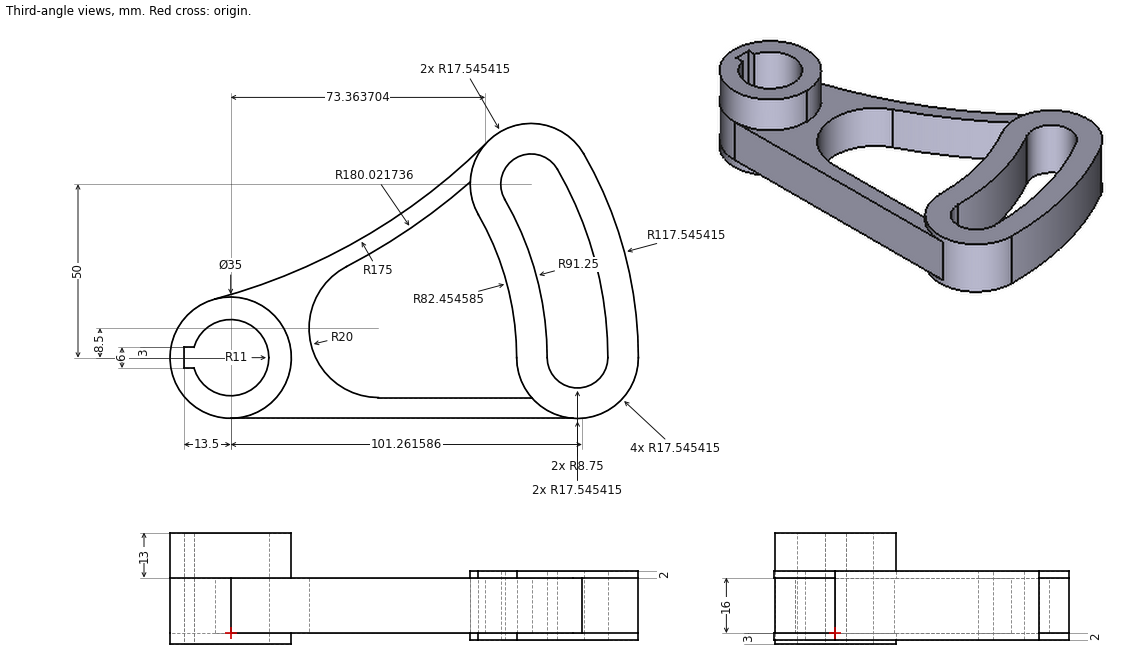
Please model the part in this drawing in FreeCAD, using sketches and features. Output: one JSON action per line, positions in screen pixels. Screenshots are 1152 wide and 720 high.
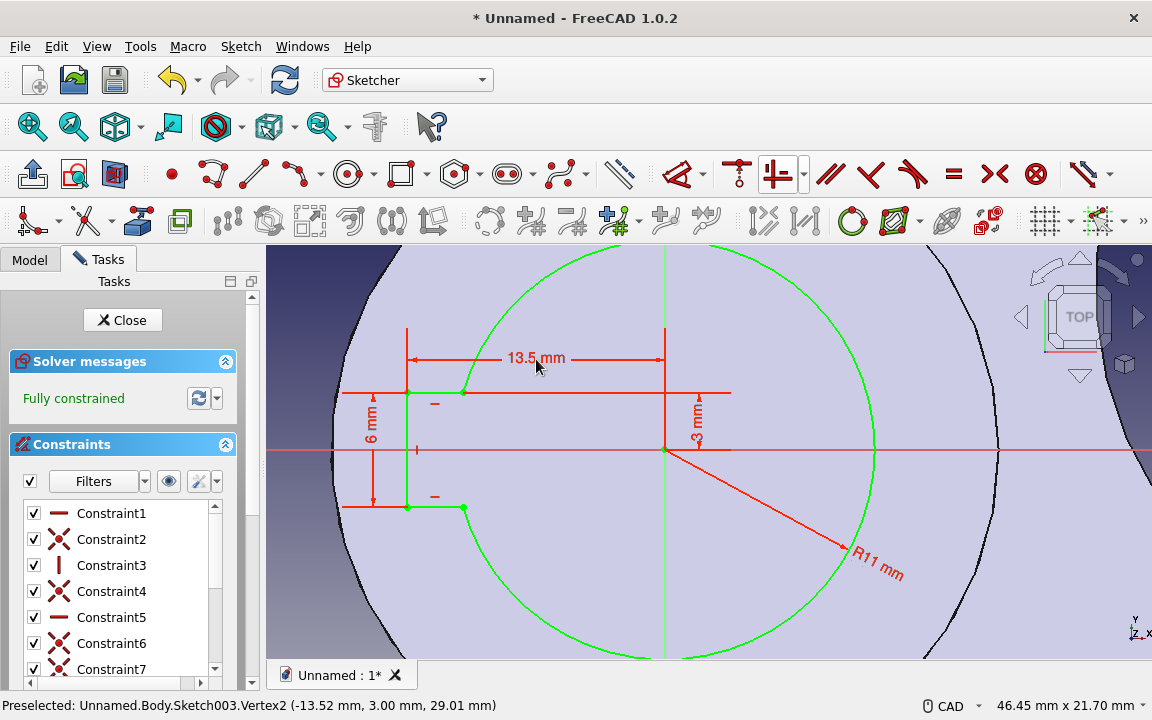
{"action": "left_click", "coordinate": [123, 320]}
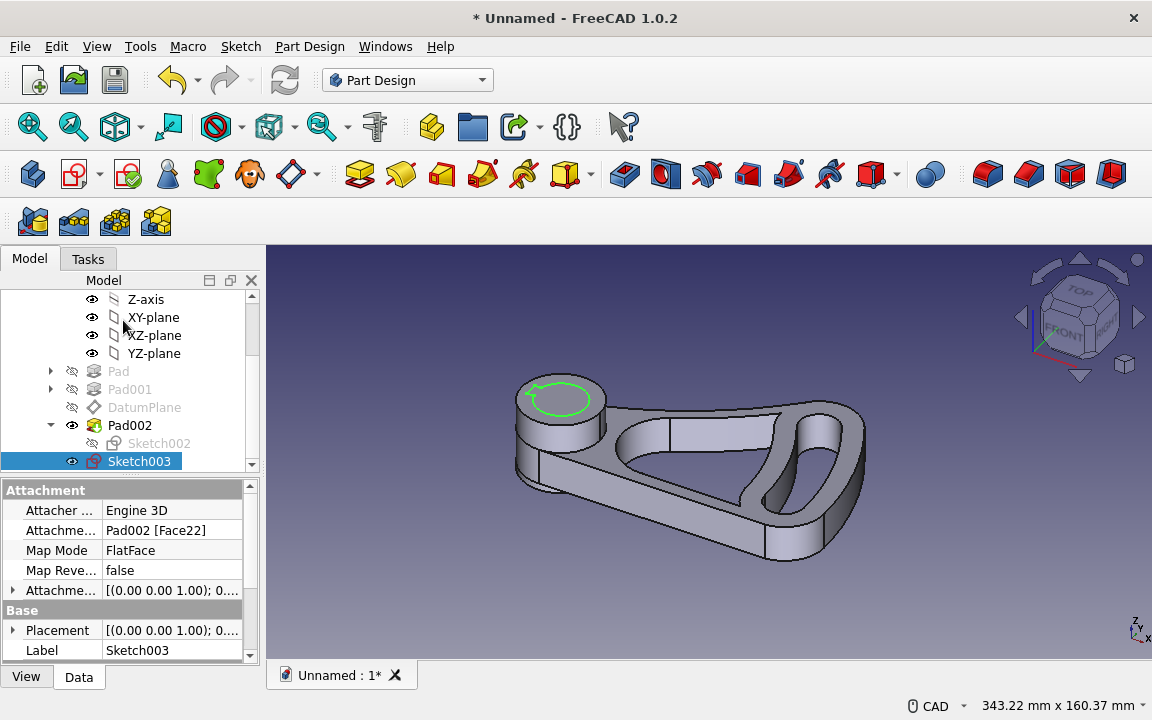
{"action": "left_click", "coordinate": [625, 174]}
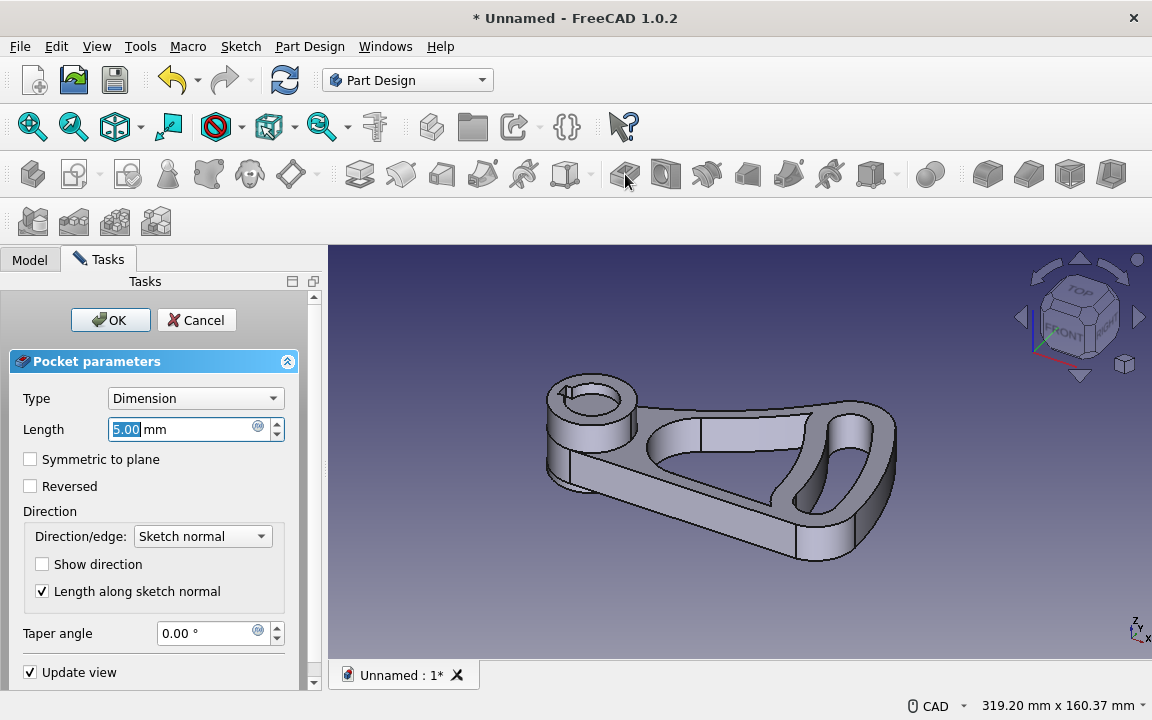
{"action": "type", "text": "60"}
{"action": "key", "text": "Tab"}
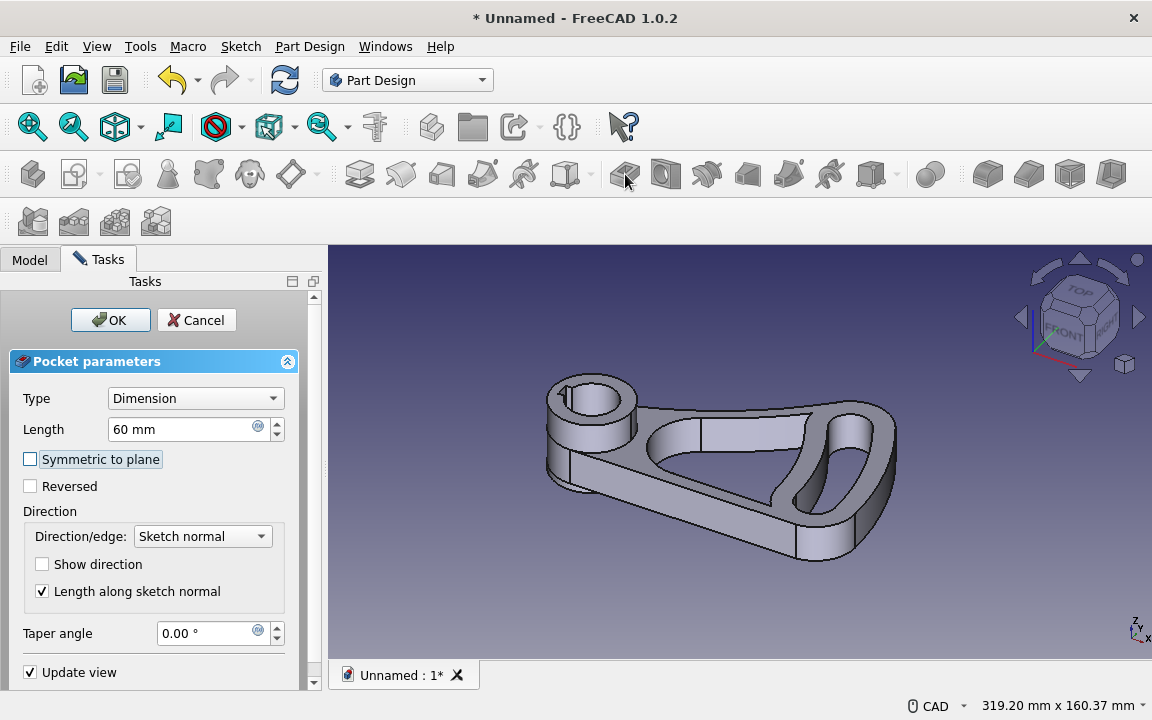
{"action": "left_click", "coordinate": [111, 320]}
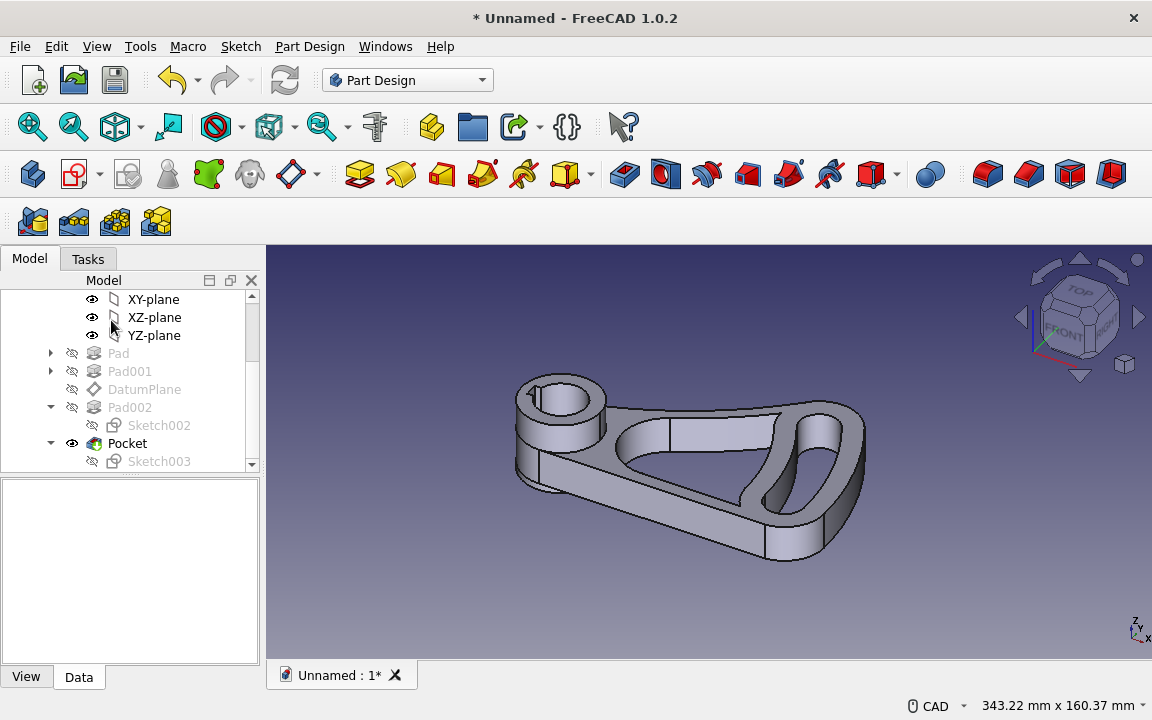
{"action": "left_click", "coordinate": [595, 457]}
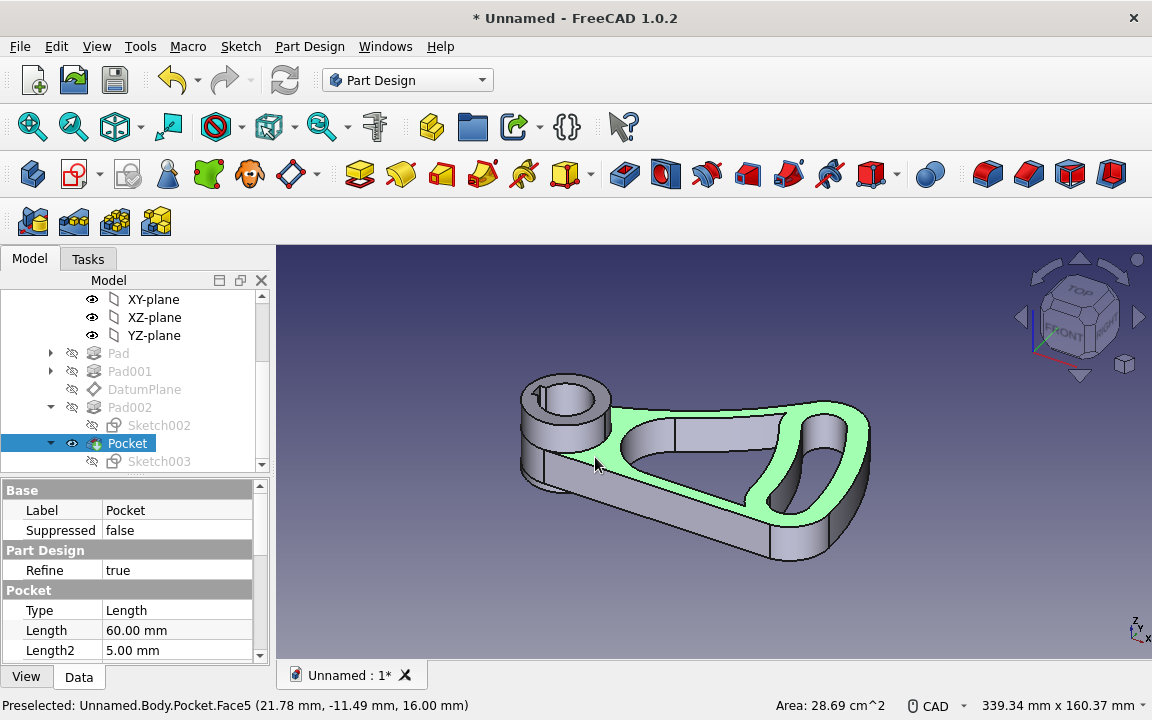
{"action": "left_click", "coordinate": [74, 174]}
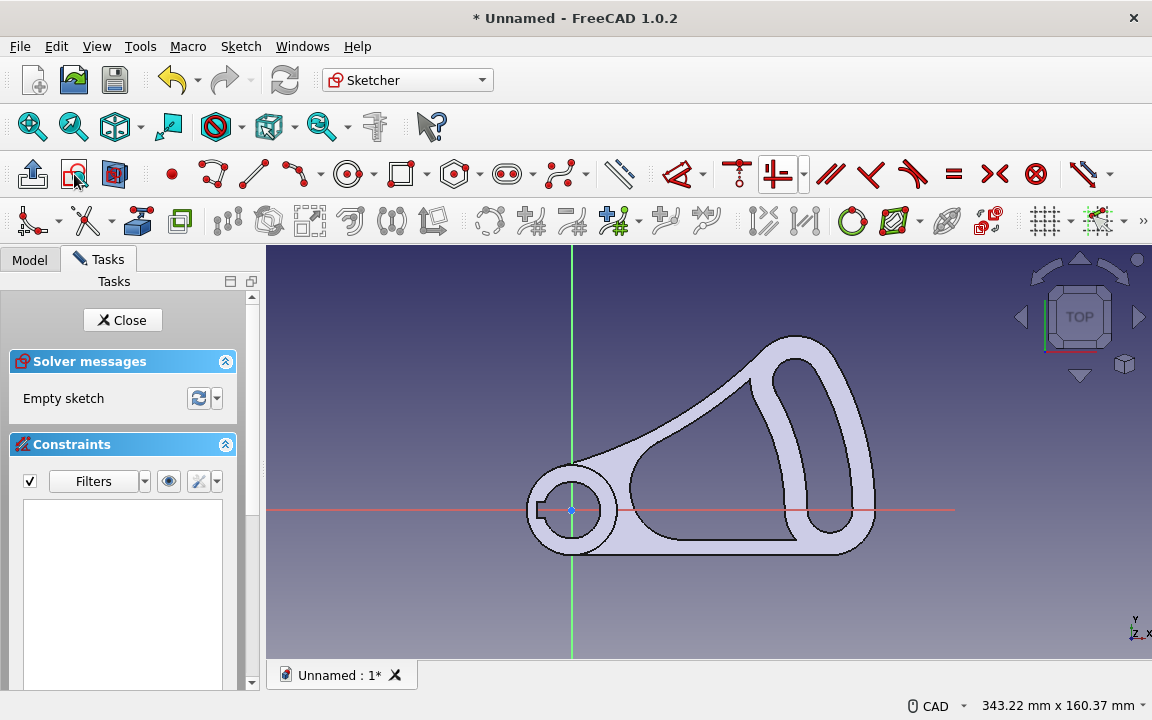
{"action": "left_click", "coordinate": [294, 174]}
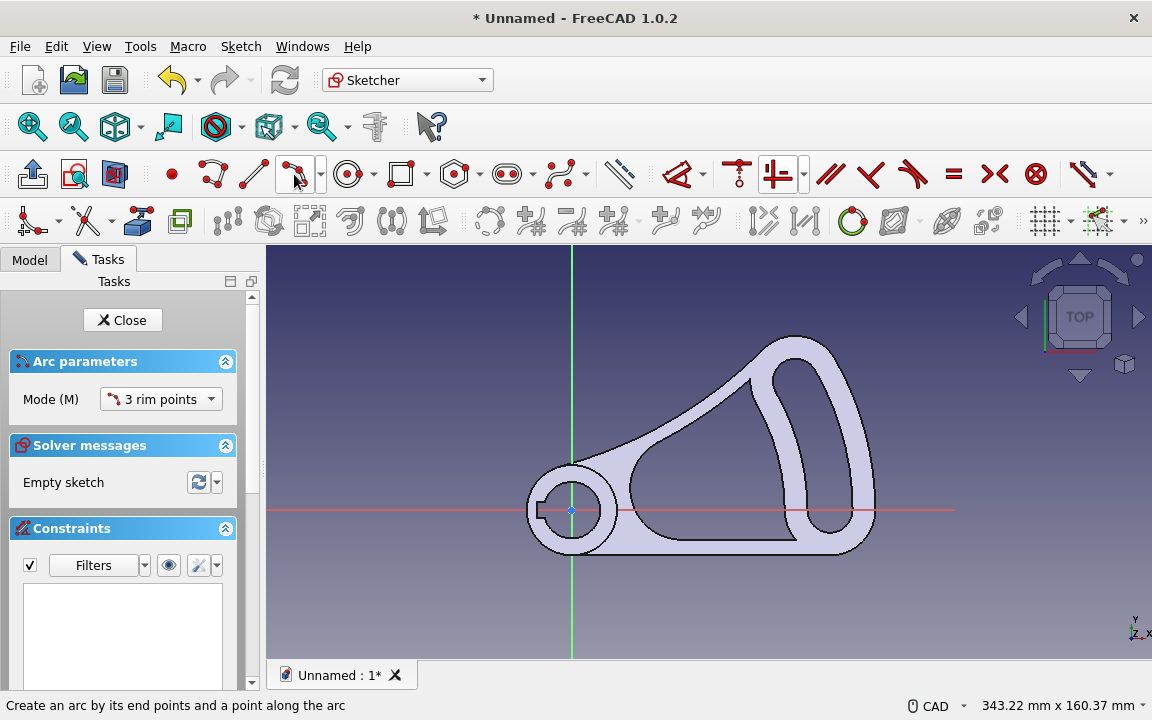
{"action": "left_click", "coordinate": [785, 510]}
{"action": "left_click", "coordinate": [875, 510]}
{"action": "left_click", "coordinate": [830, 556]}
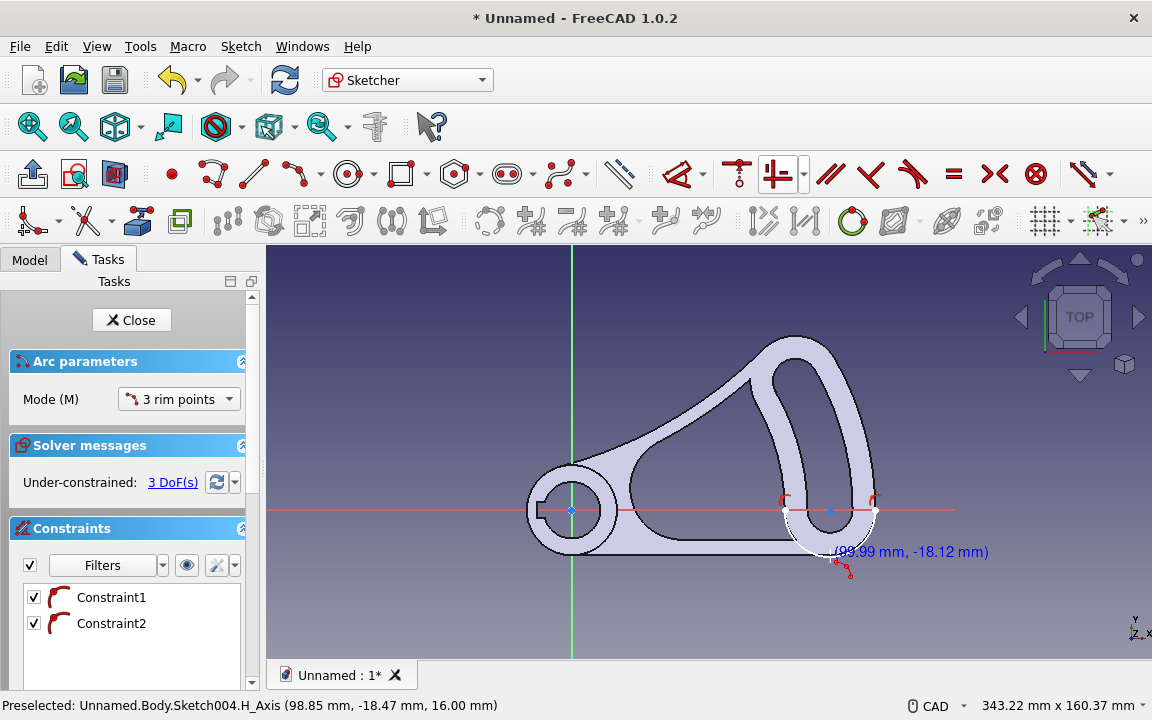
{"action": "left_click", "coordinate": [875, 510]}
{"action": "left_click", "coordinate": [835, 359]}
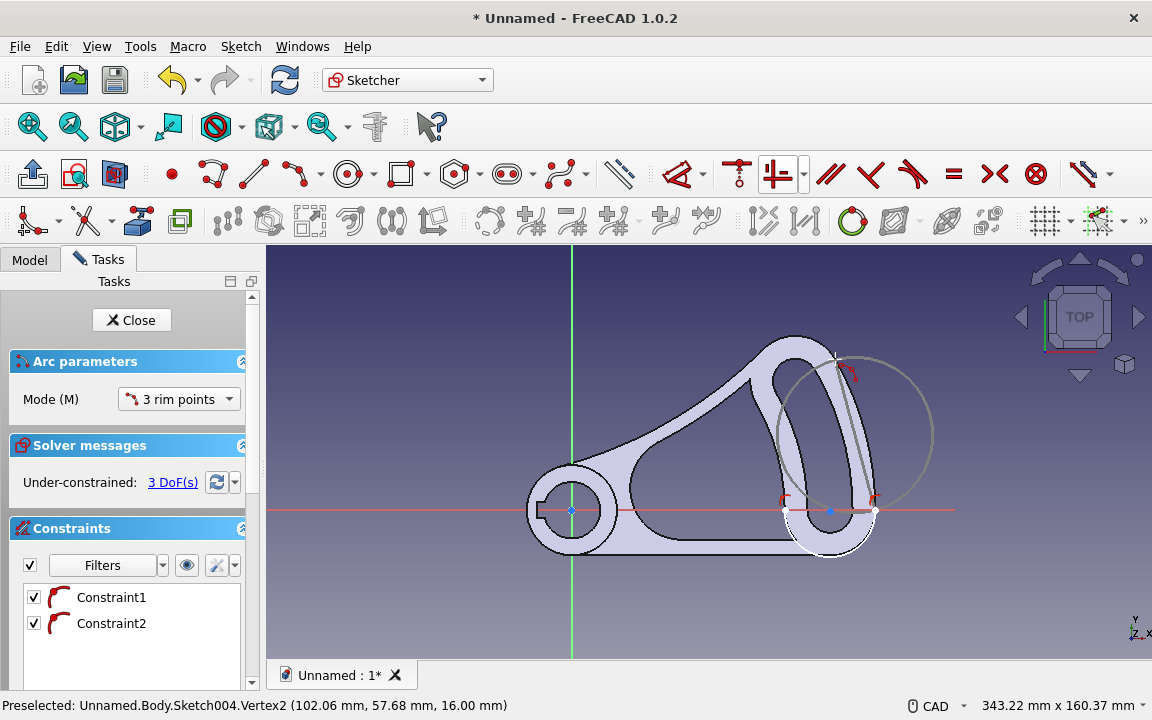
{"action": "scroll", "coordinate": [865, 432], "scroll_direction": "up", "scroll_amount": 3}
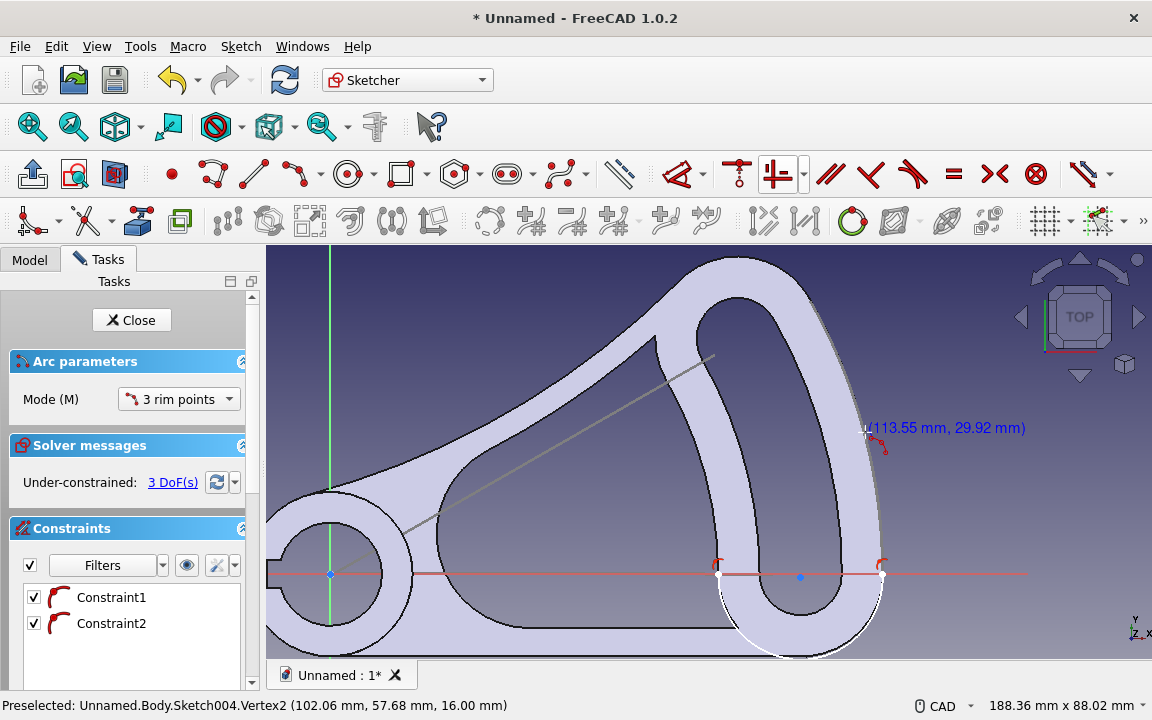
{"action": "left_click", "coordinate": [864, 431]}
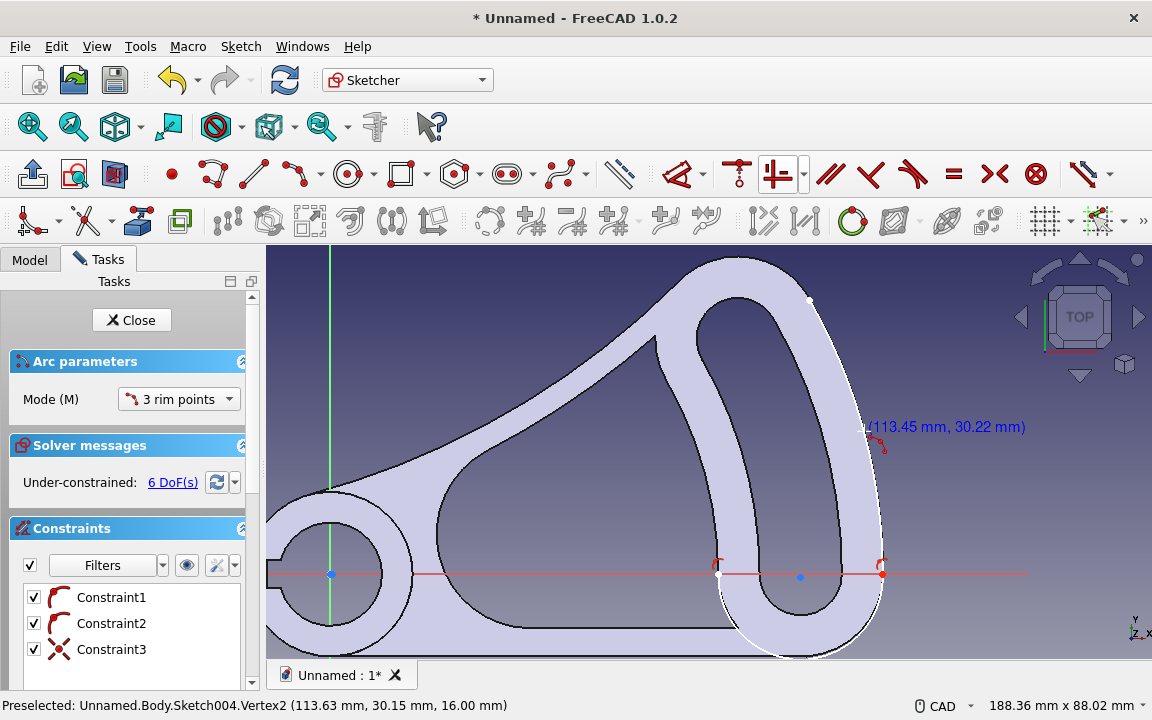
{"action": "left_click", "coordinate": [810, 300]}
{"action": "left_click", "coordinate": [666, 380]}